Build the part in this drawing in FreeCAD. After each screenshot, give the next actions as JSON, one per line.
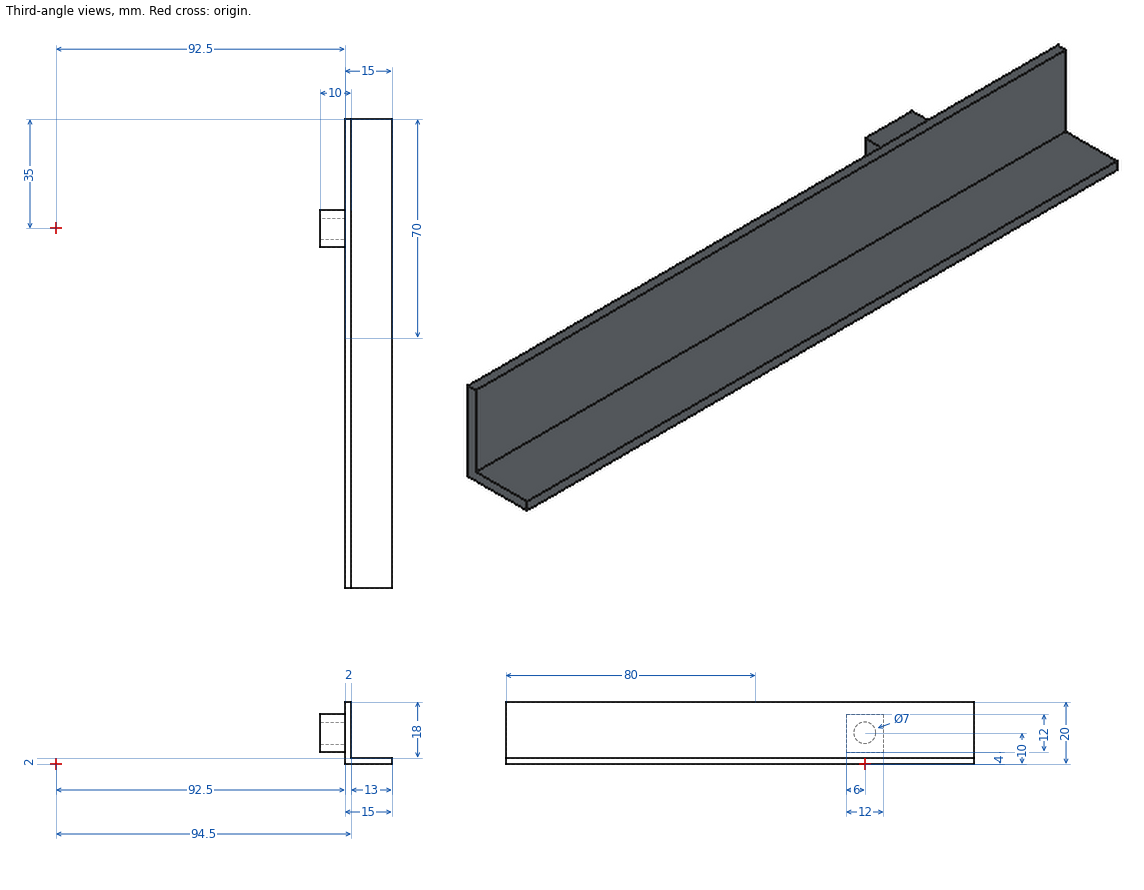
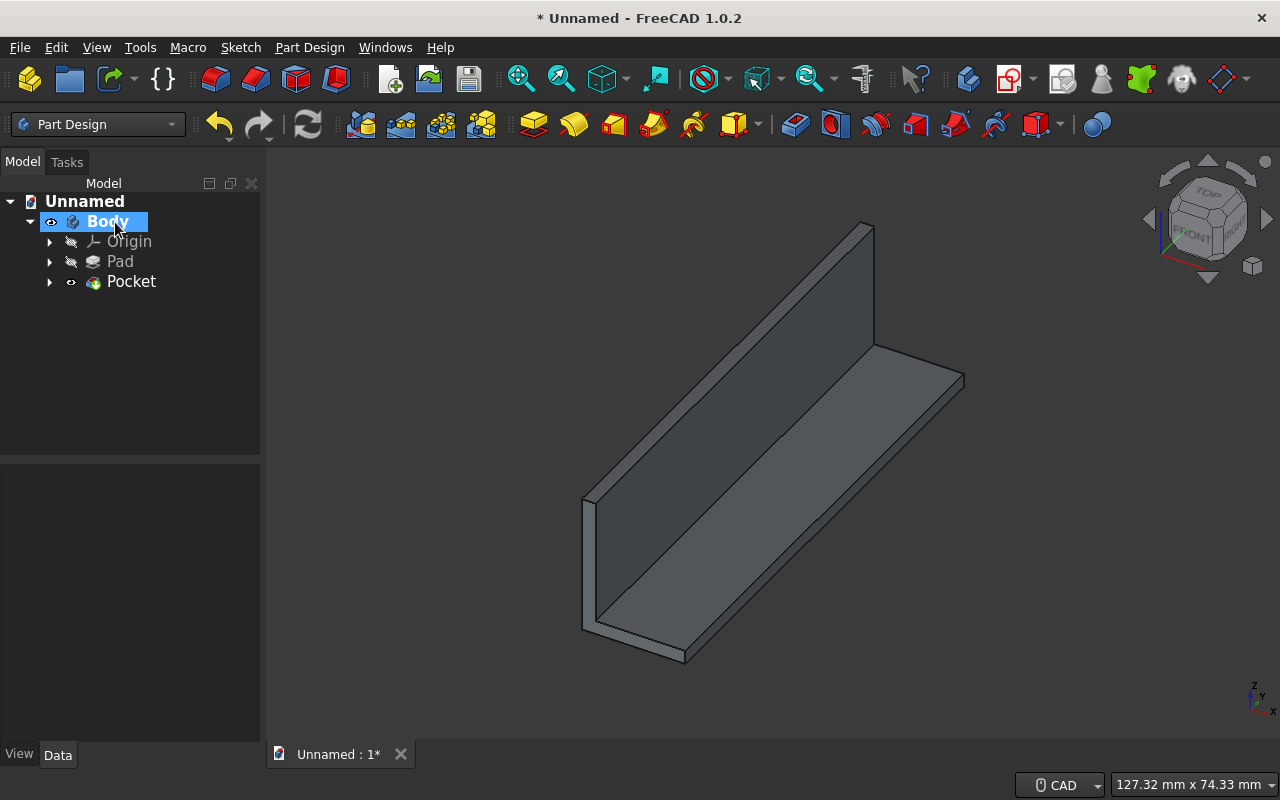
{"action": "key", "text": "0"}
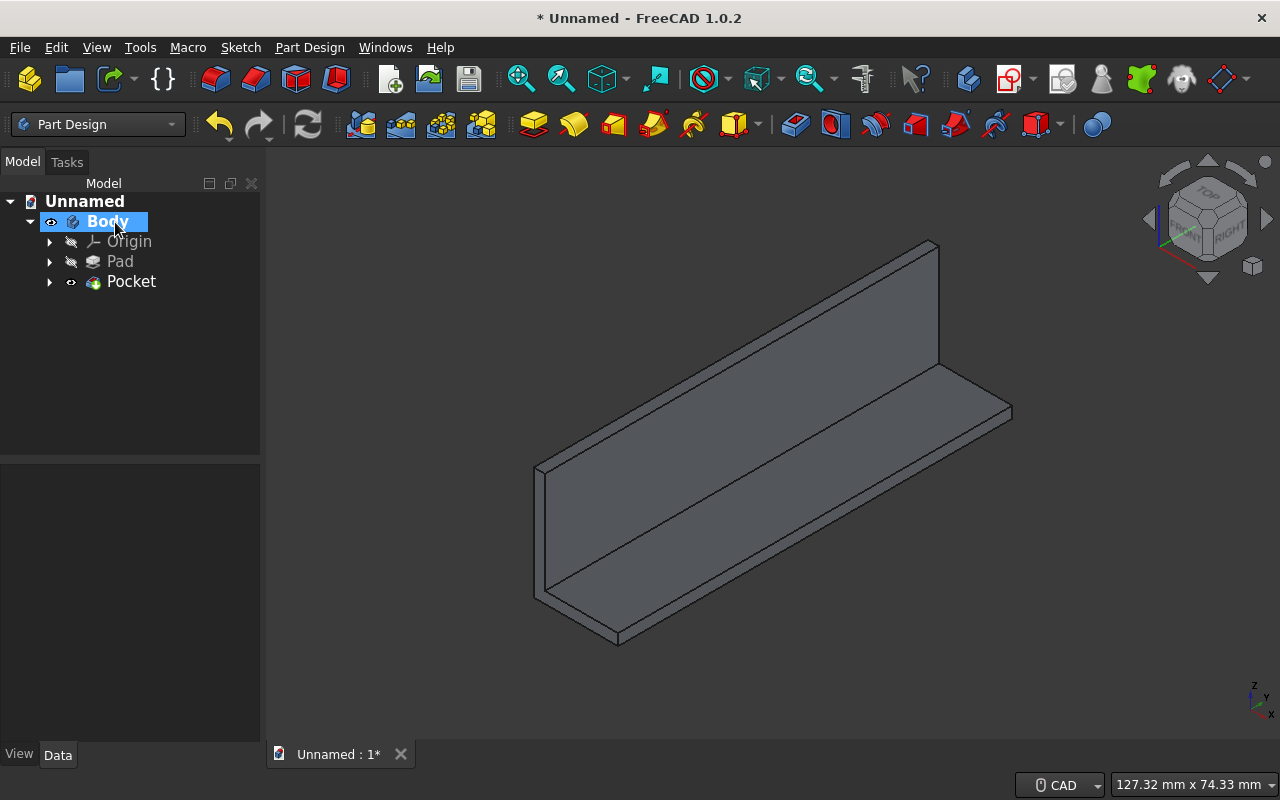
{"action": "key", "text": "1"}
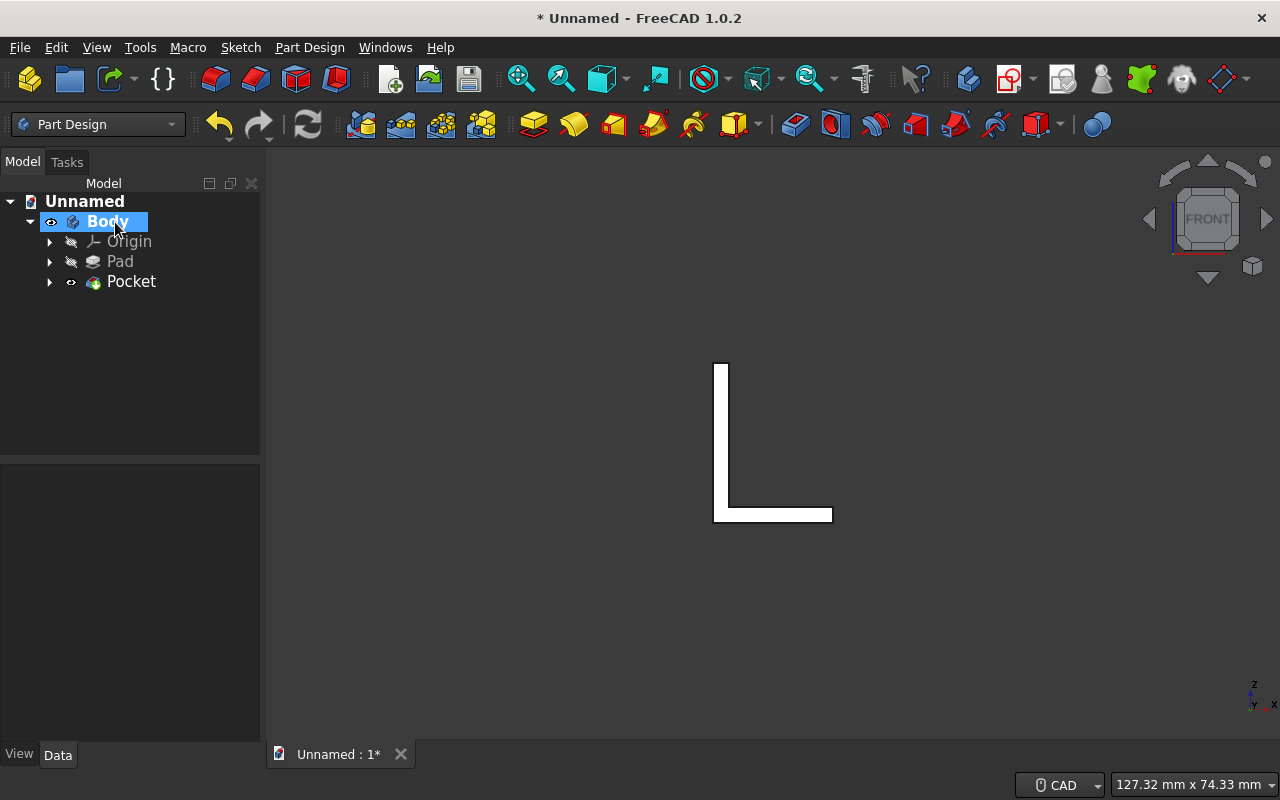
{"action": "left_click", "coordinate": [522, 80]}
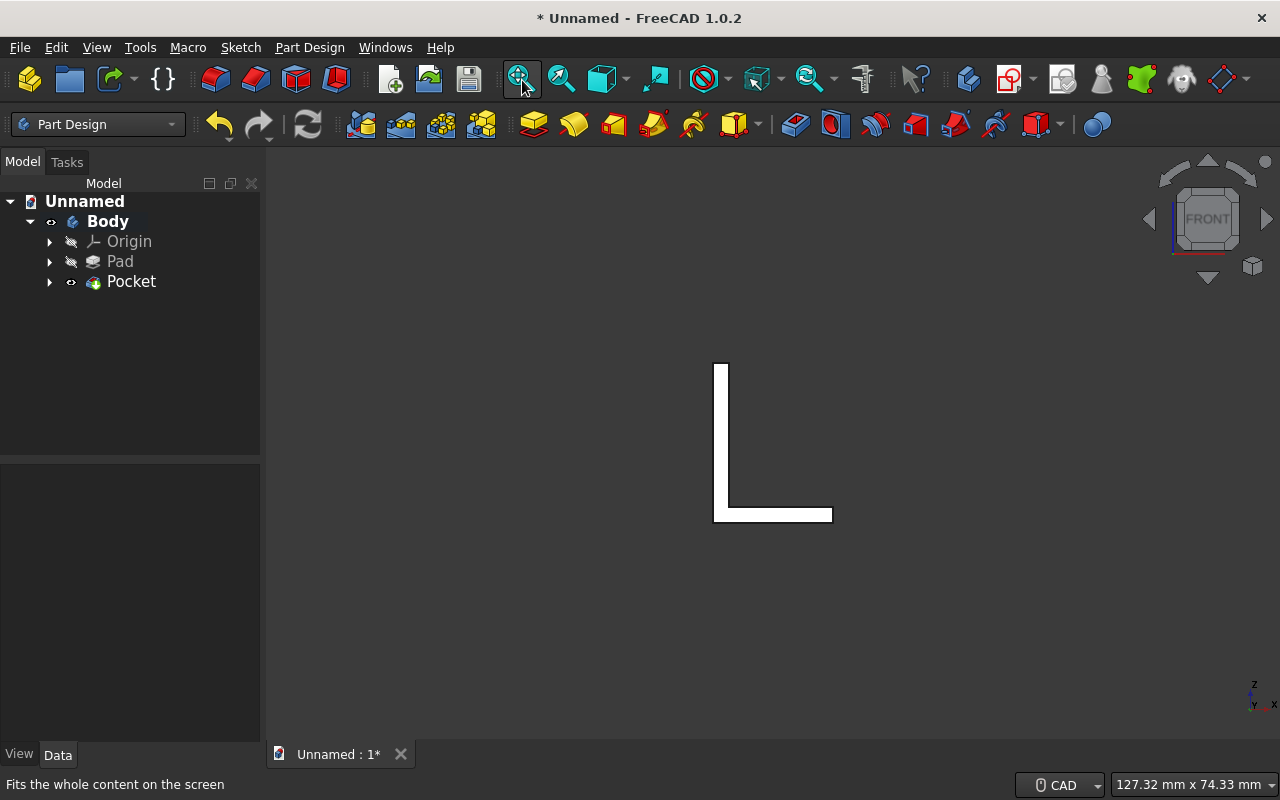
{"action": "key", "text": "2"}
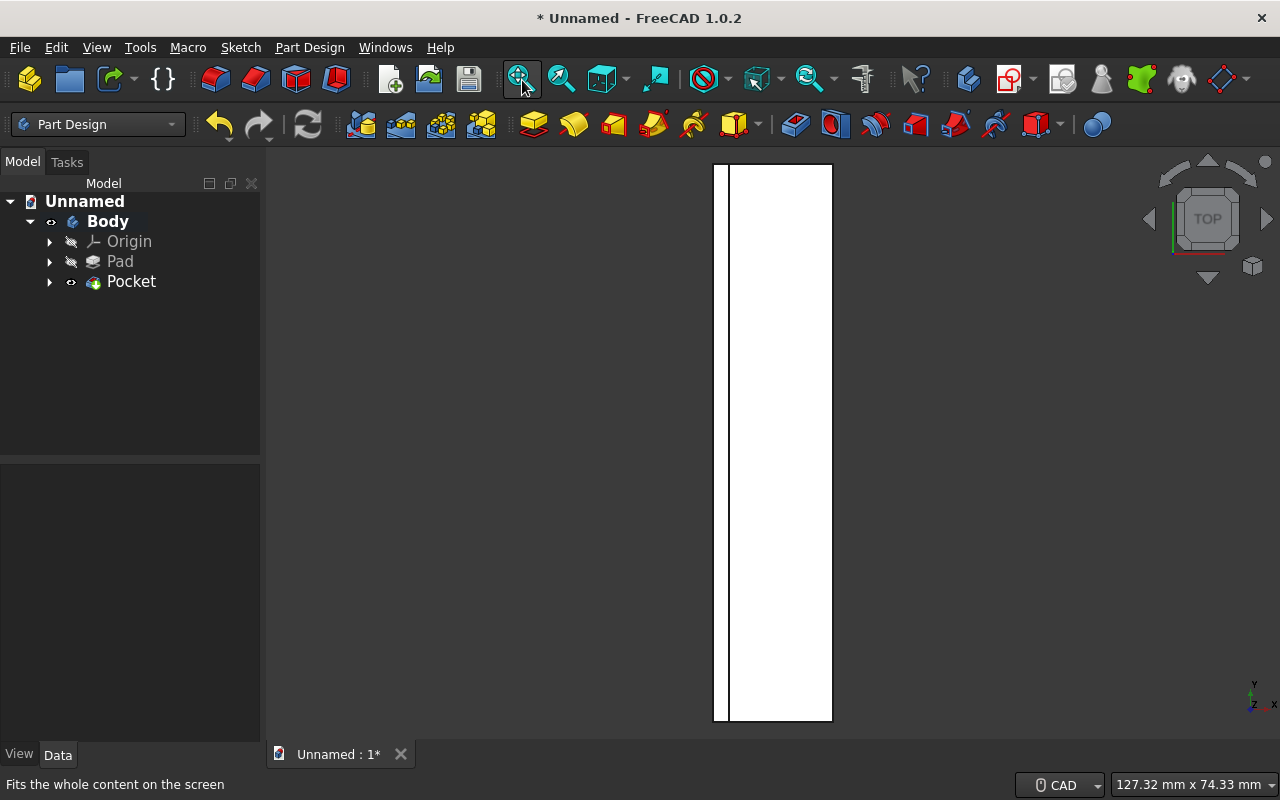
{"action": "left_click", "coordinate": [50, 242]}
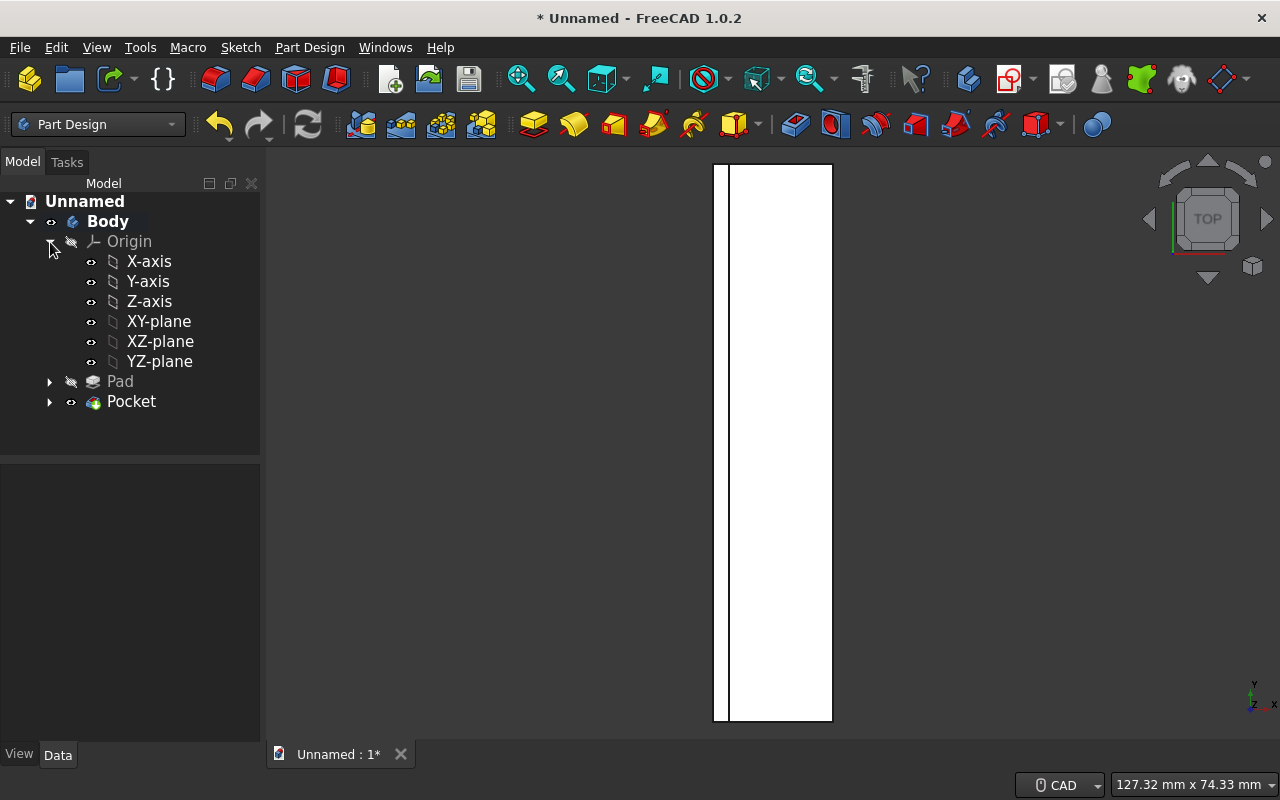
{"action": "left_click", "coordinate": [136, 342]}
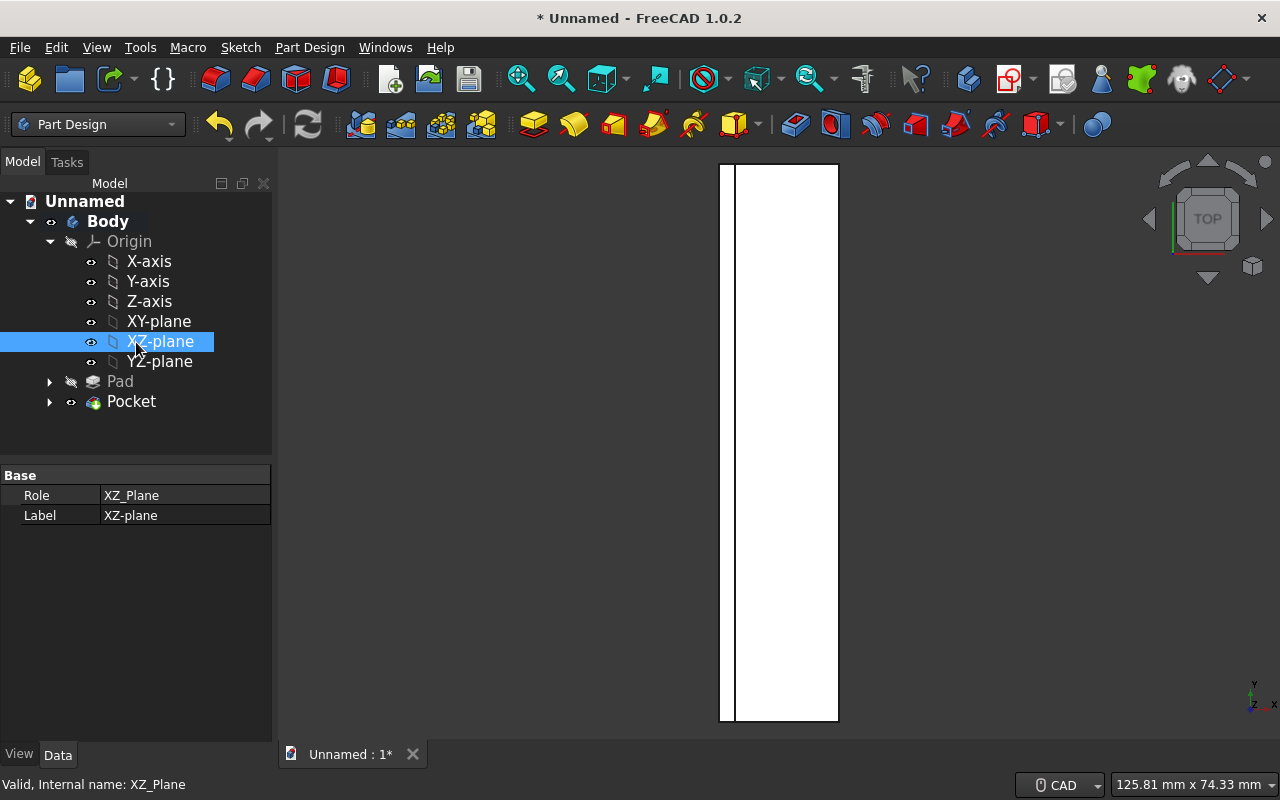
{"action": "left_click", "coordinate": [1222, 80]}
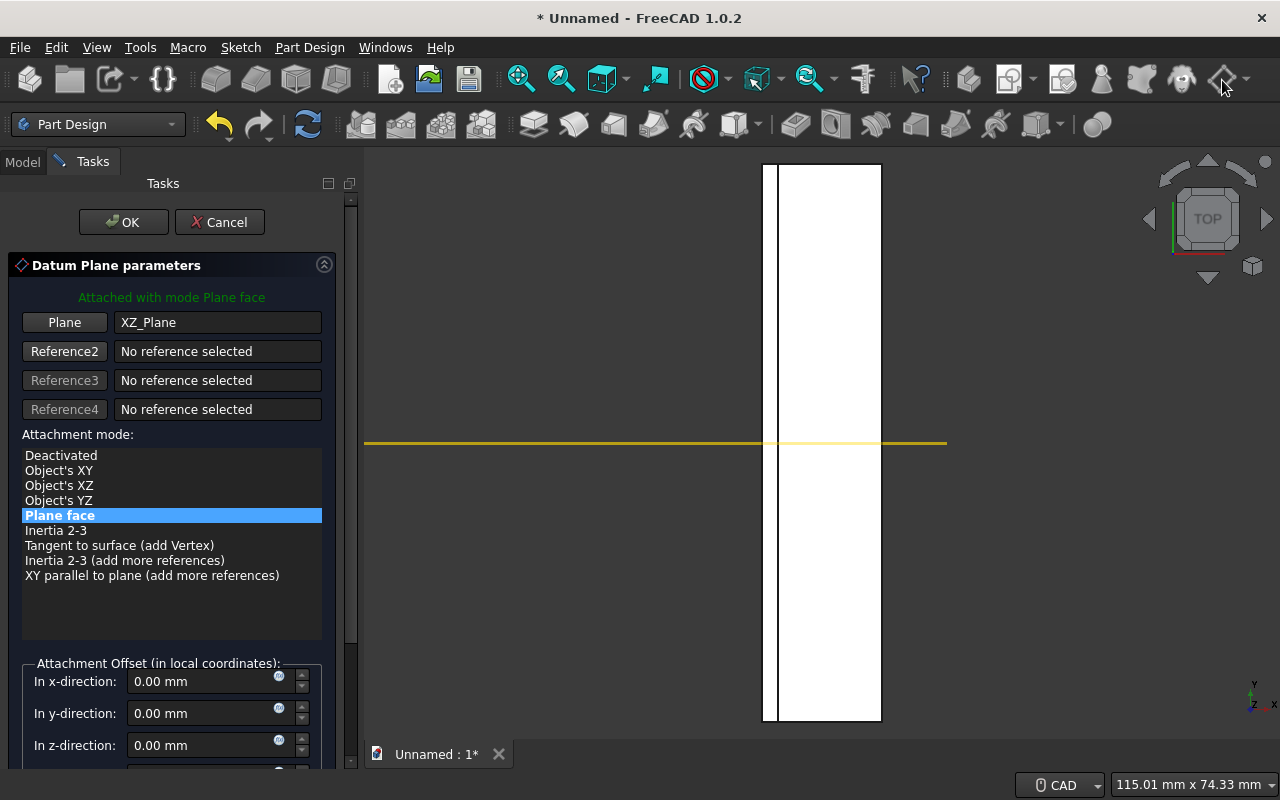
{"action": "triple_click", "coordinate": [210, 745]}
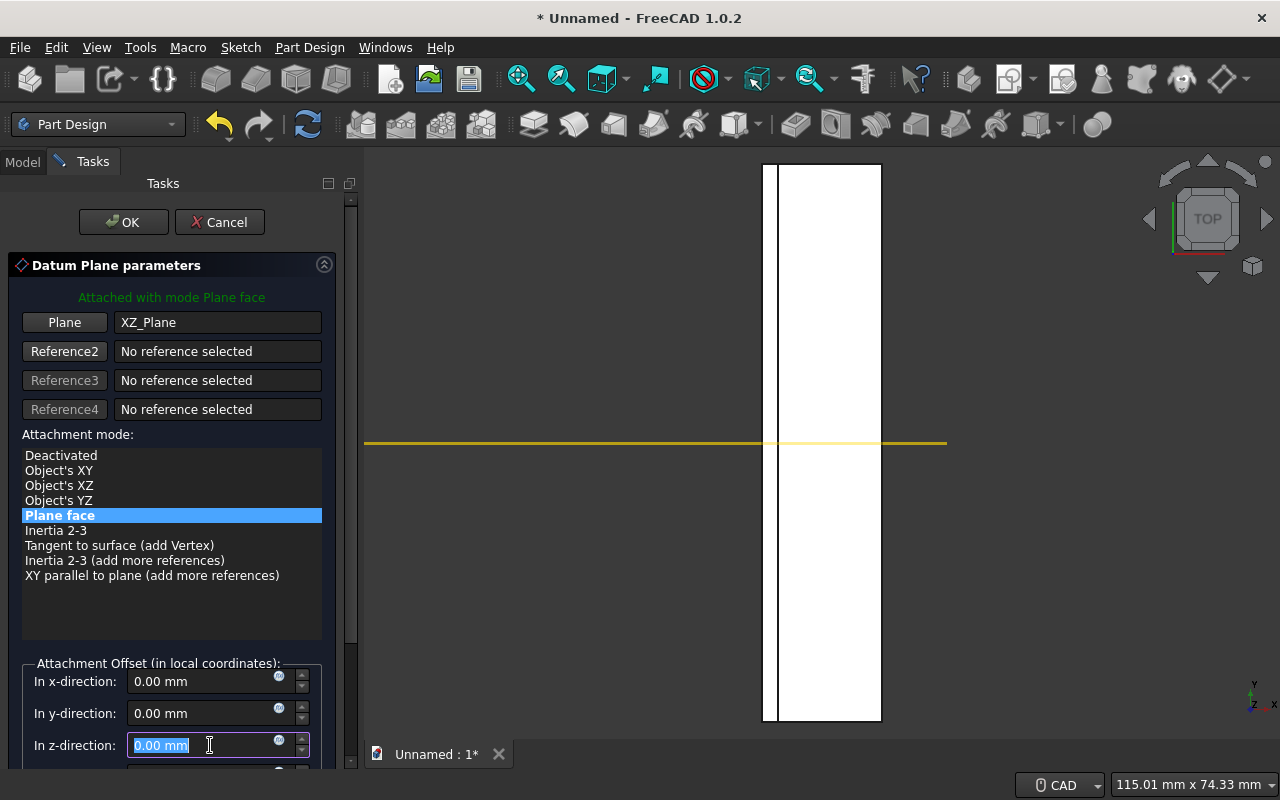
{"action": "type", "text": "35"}
{"action": "key", "text": "Tab"}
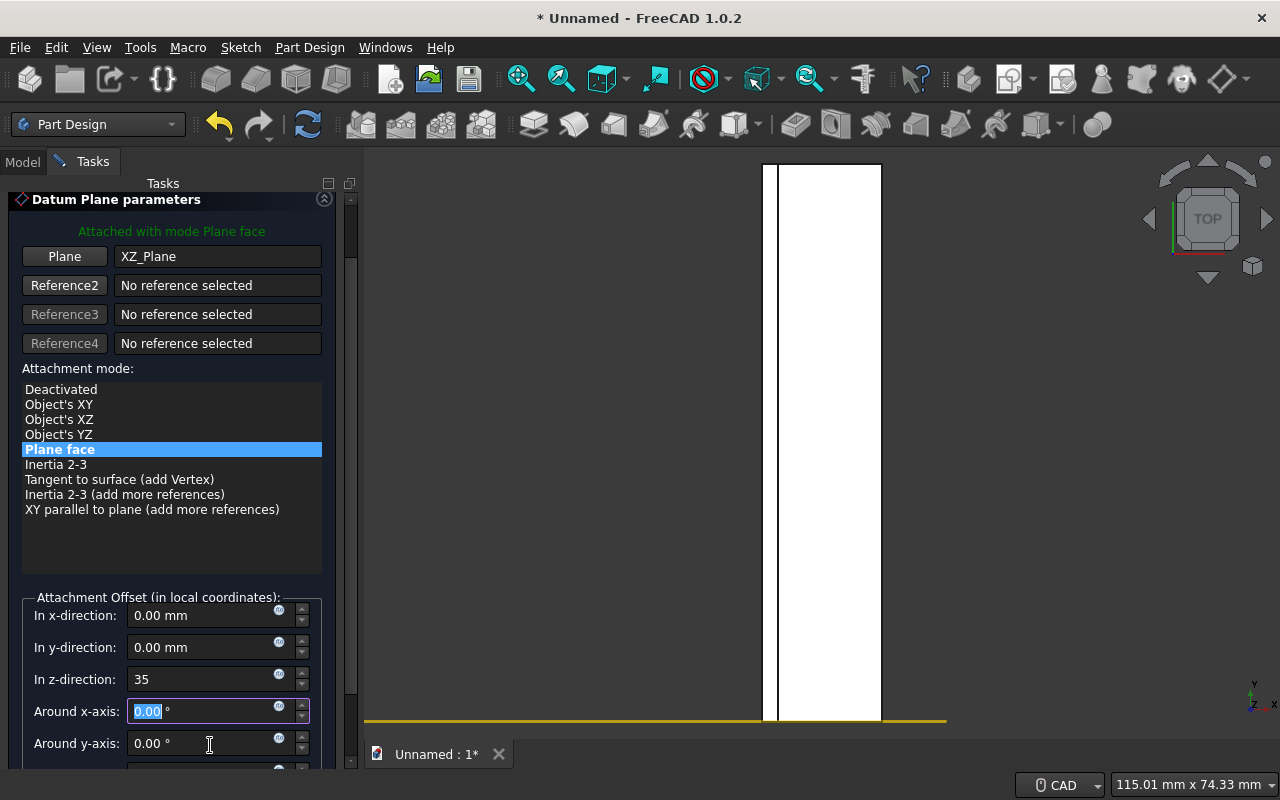
{"action": "scroll", "coordinate": [351, 480], "scroll_direction": "up", "scroll_amount": 2}